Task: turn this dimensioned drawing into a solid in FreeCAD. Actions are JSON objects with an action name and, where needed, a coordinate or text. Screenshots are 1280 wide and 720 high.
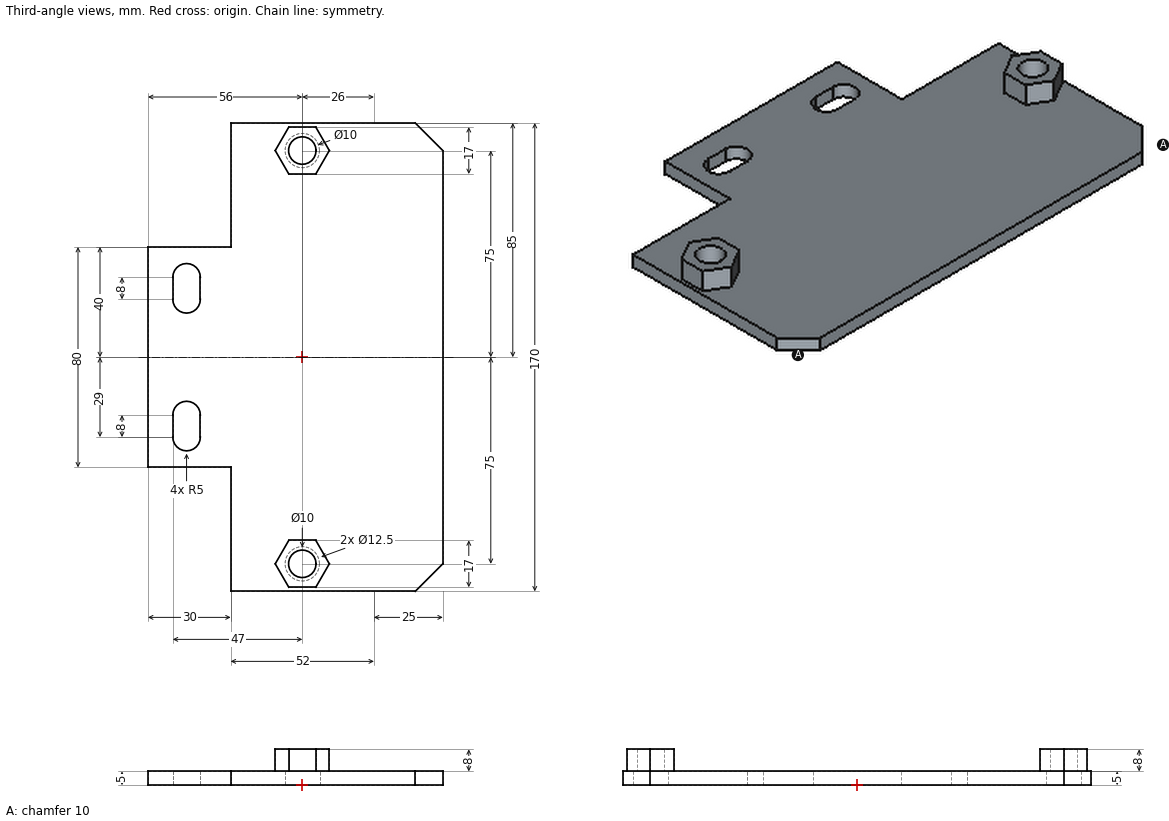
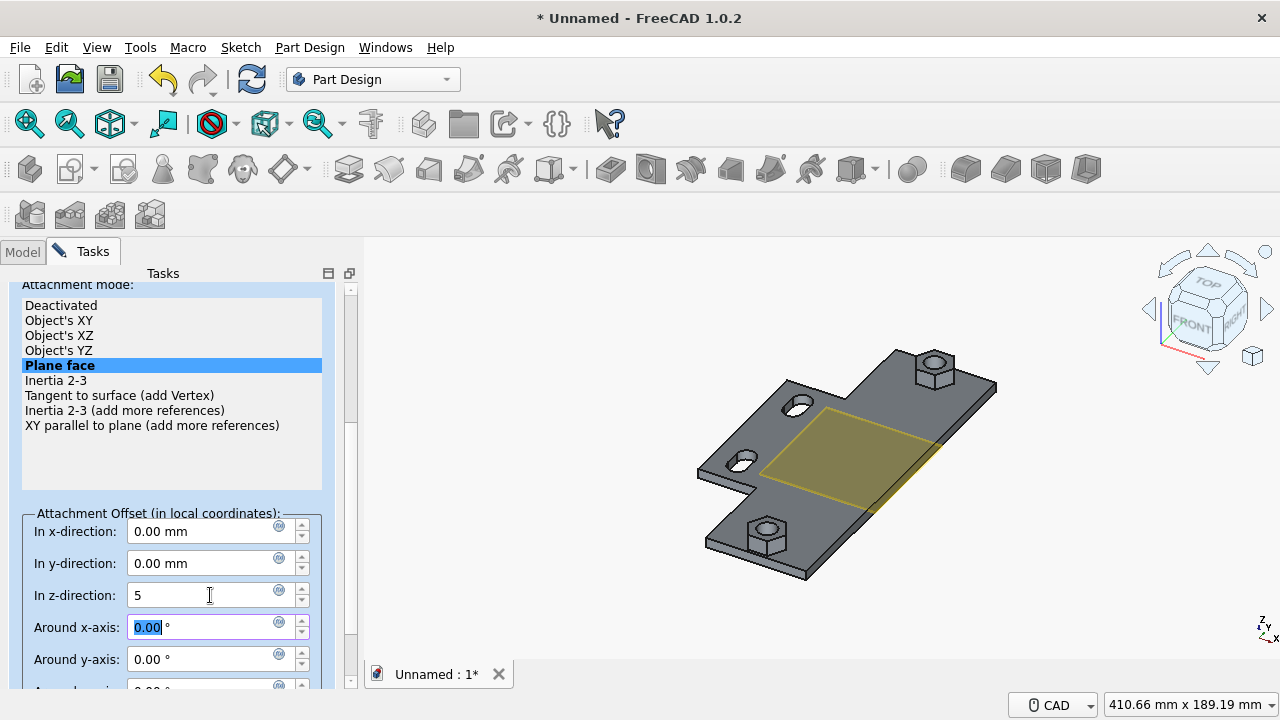
{"action": "scroll", "coordinate": [351, 486], "scroll_direction": "up", "scroll_amount": 5}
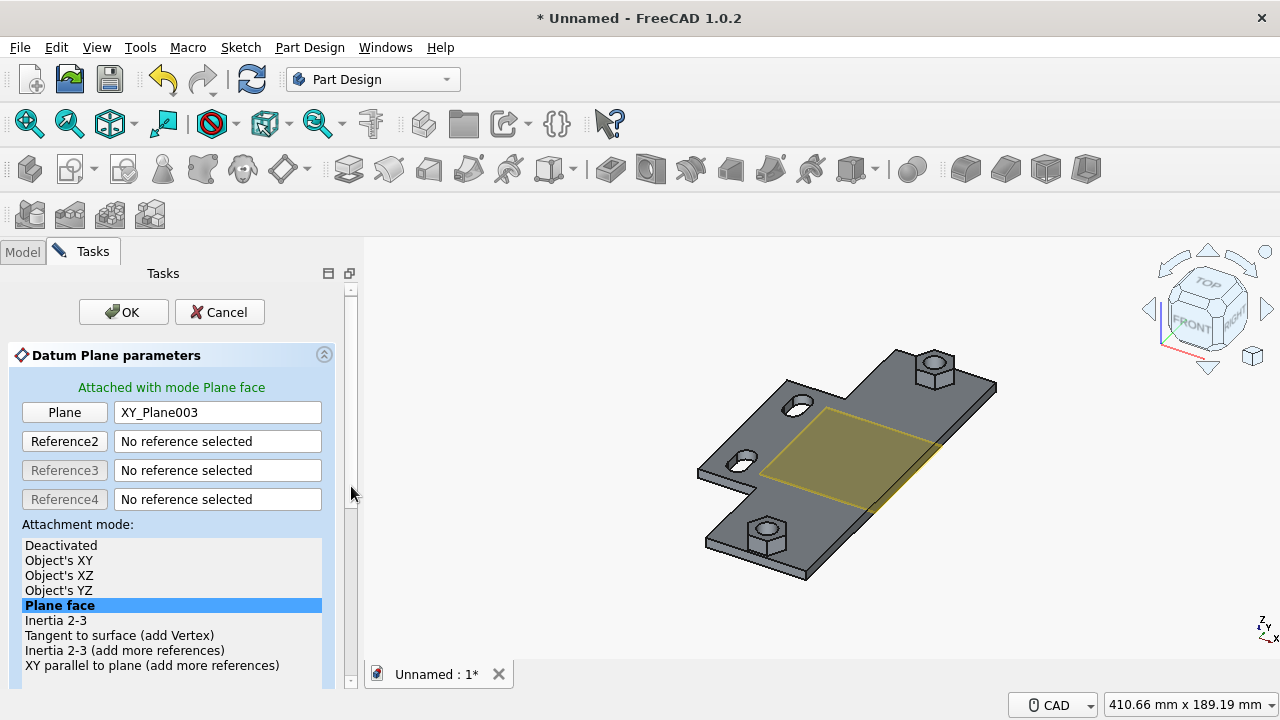
{"action": "left_click", "coordinate": [124, 312]}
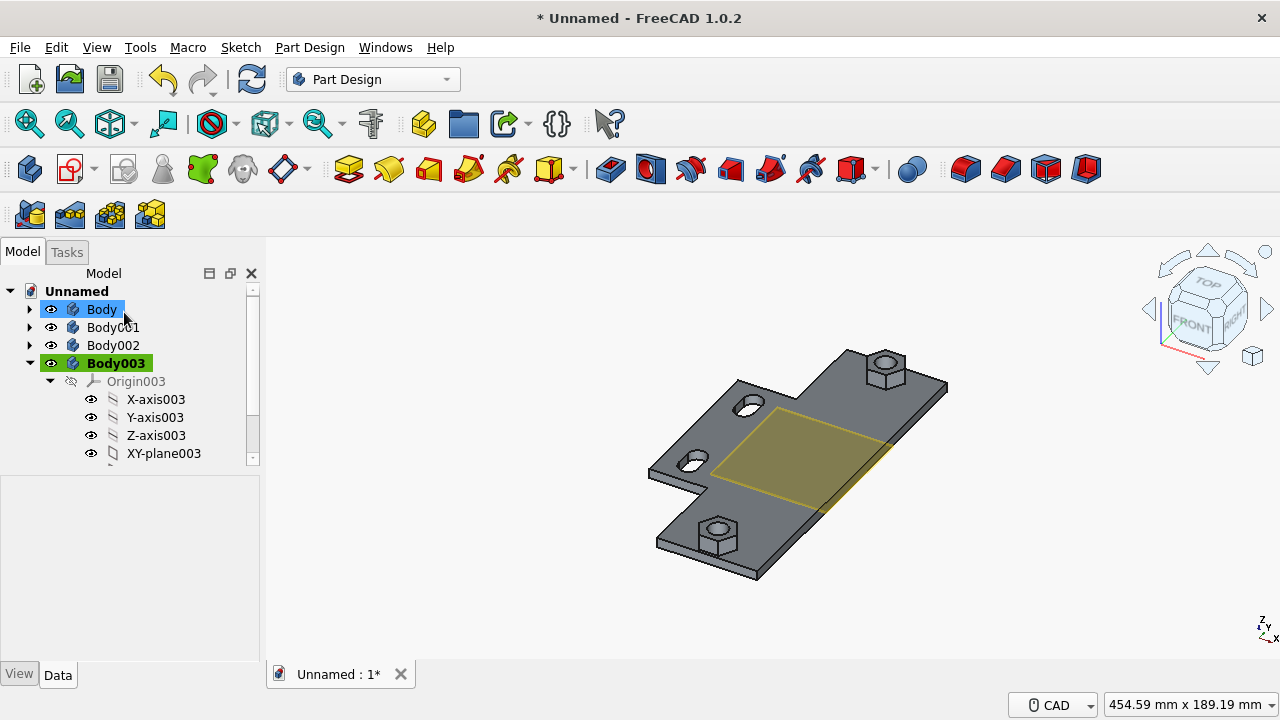
{"action": "scroll", "coordinate": [100, 377], "scroll_direction": "down", "scroll_amount": 3}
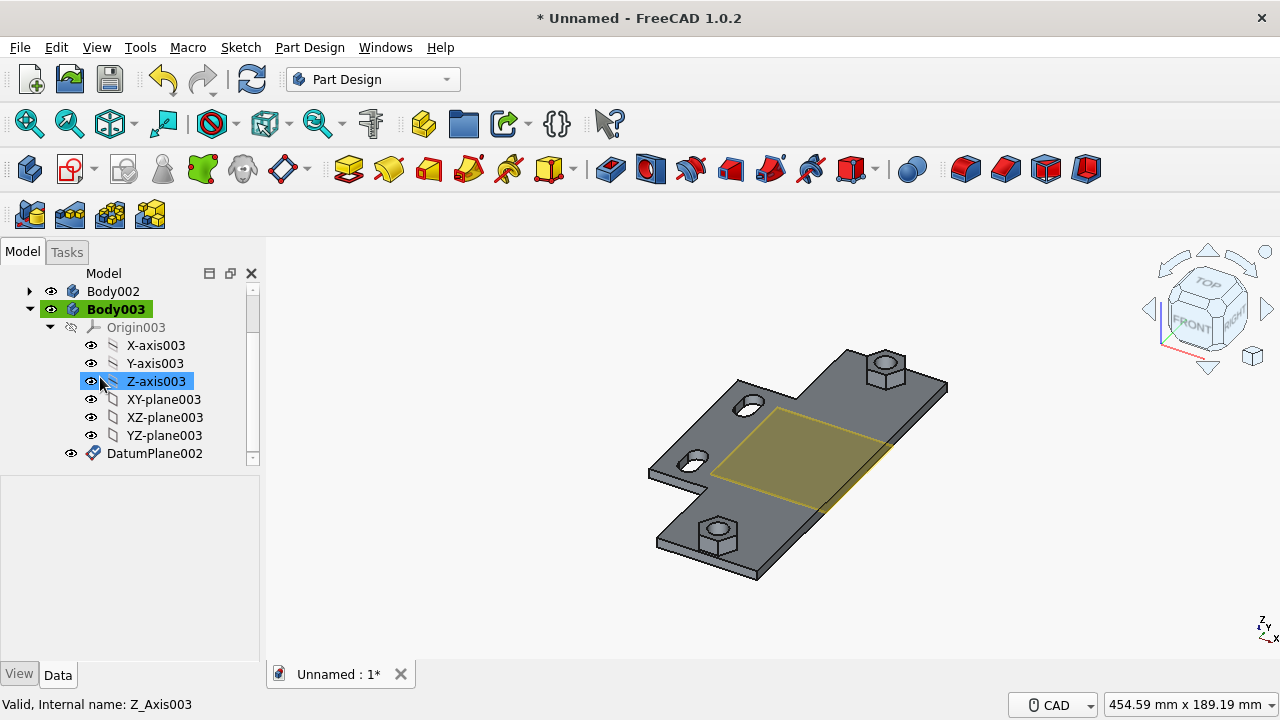
{"action": "left_click", "coordinate": [116, 453]}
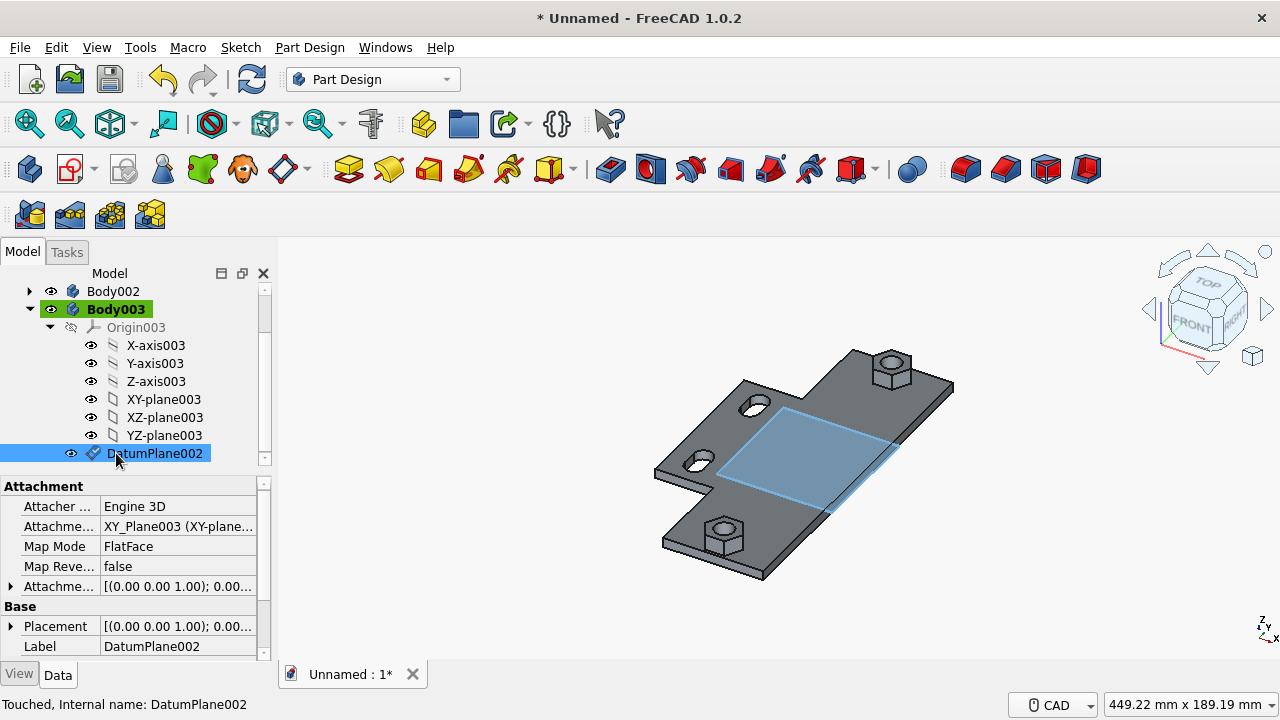
{"action": "left_click", "coordinate": [70, 170]}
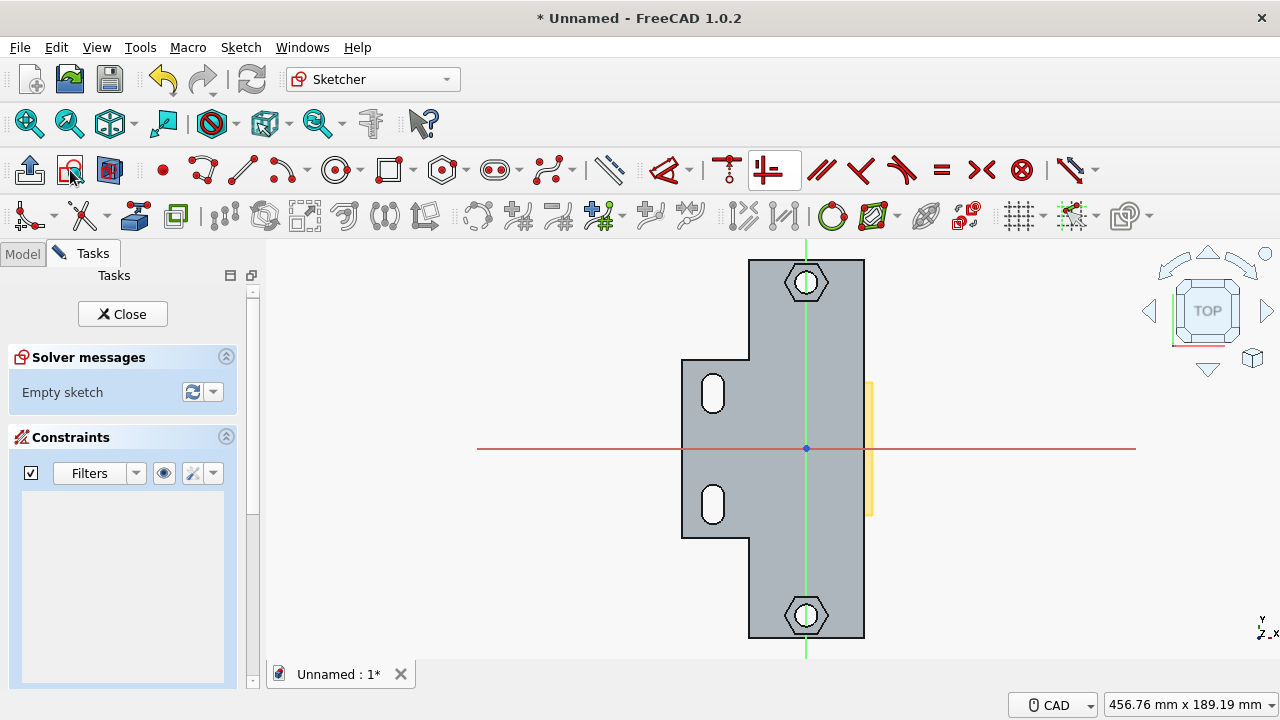
{"action": "scroll", "coordinate": [382, 449], "scroll_direction": "down", "scroll_amount": 2}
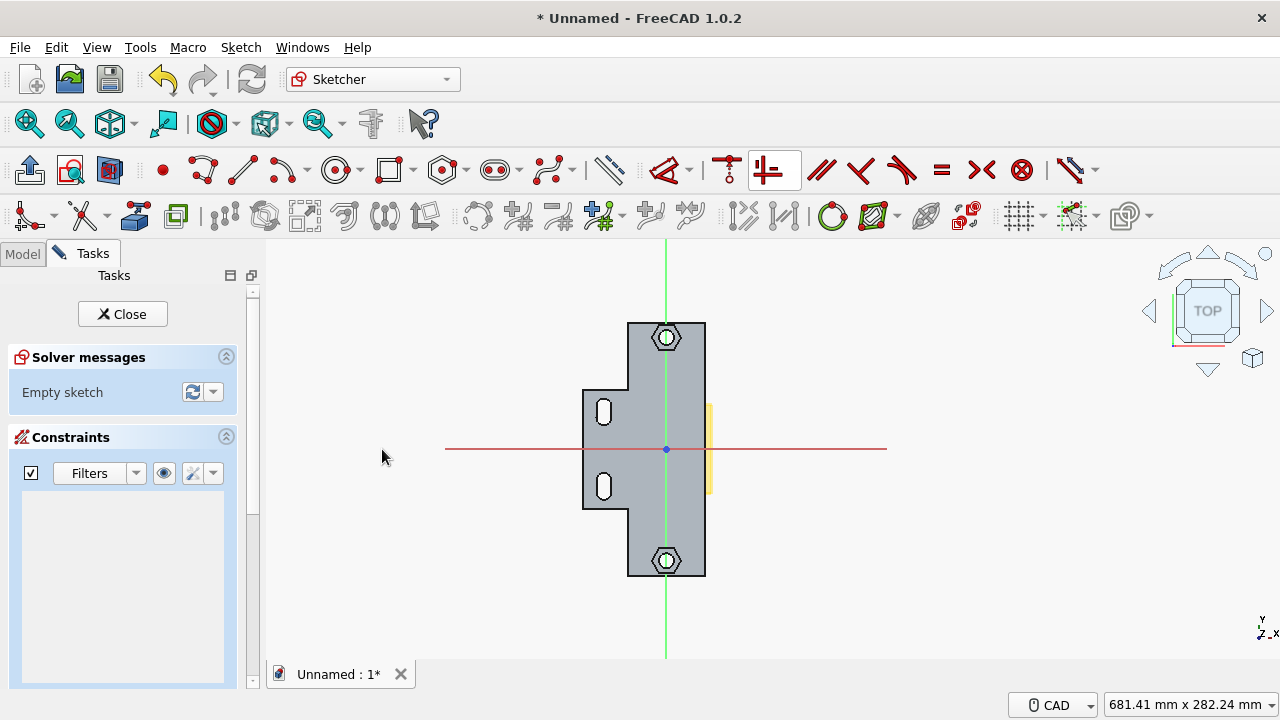
{"action": "left_click", "coordinate": [390, 170]}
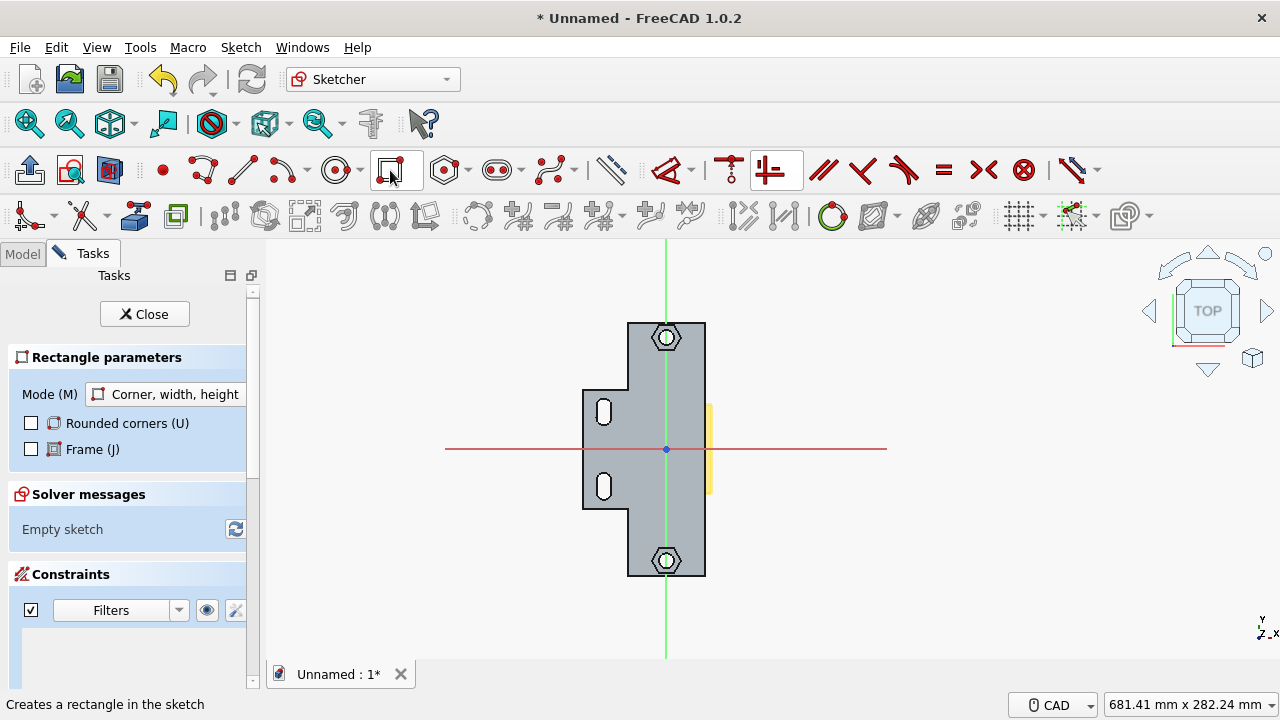
{"action": "left_click", "coordinate": [705, 323]}
{"action": "left_click", "coordinate": [742, 576]}
{"action": "key", "text": "Escape"}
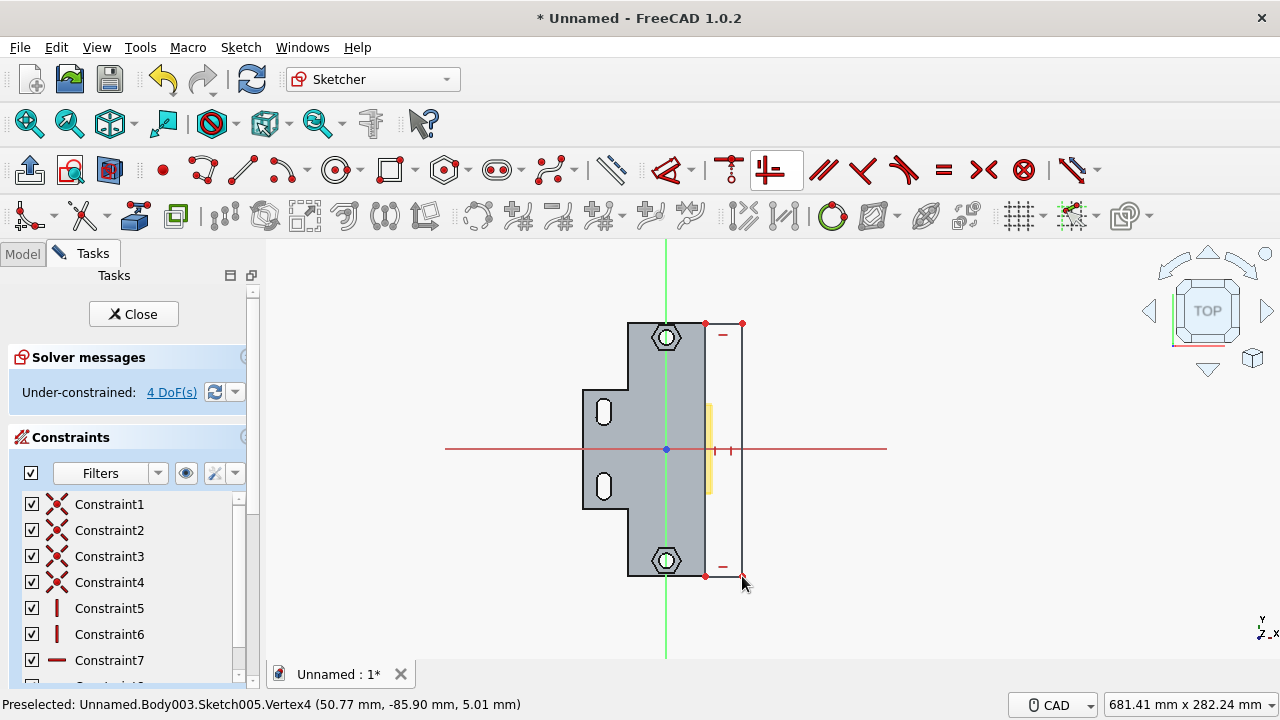
{"action": "left_click", "coordinate": [666, 170]}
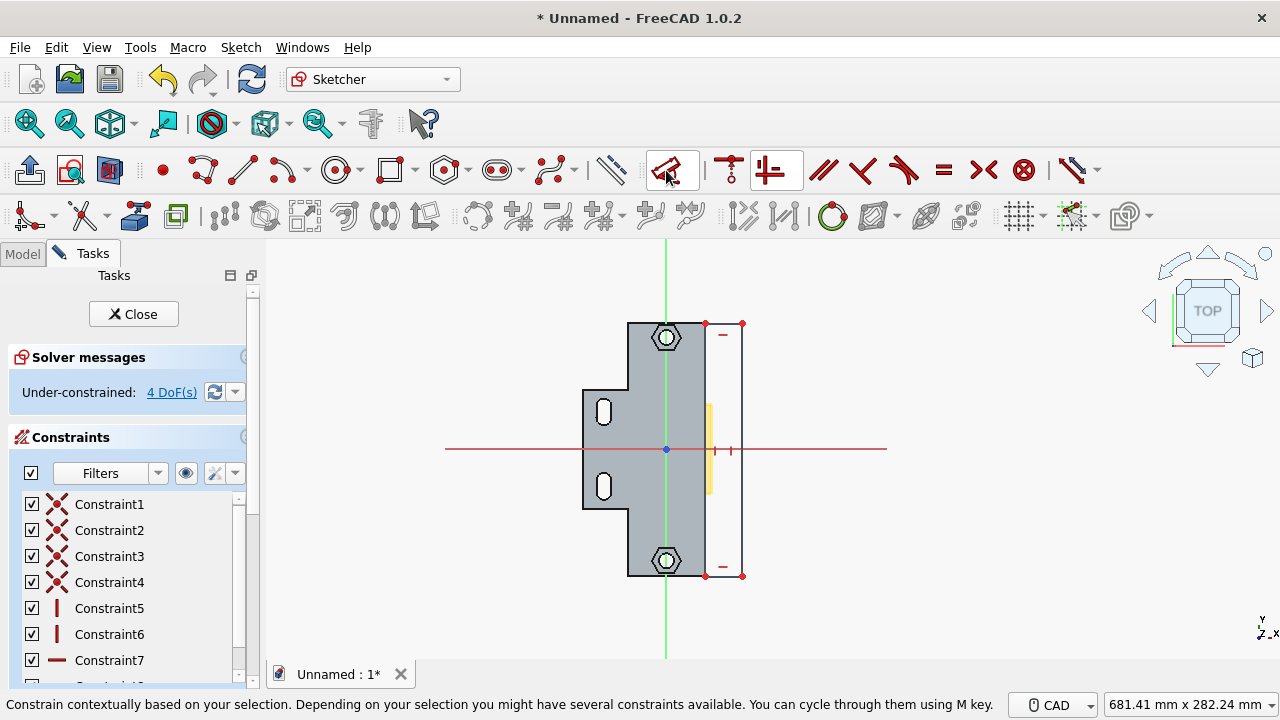
{"action": "scroll", "coordinate": [716, 577], "scroll_direction": "up", "scroll_amount": 2}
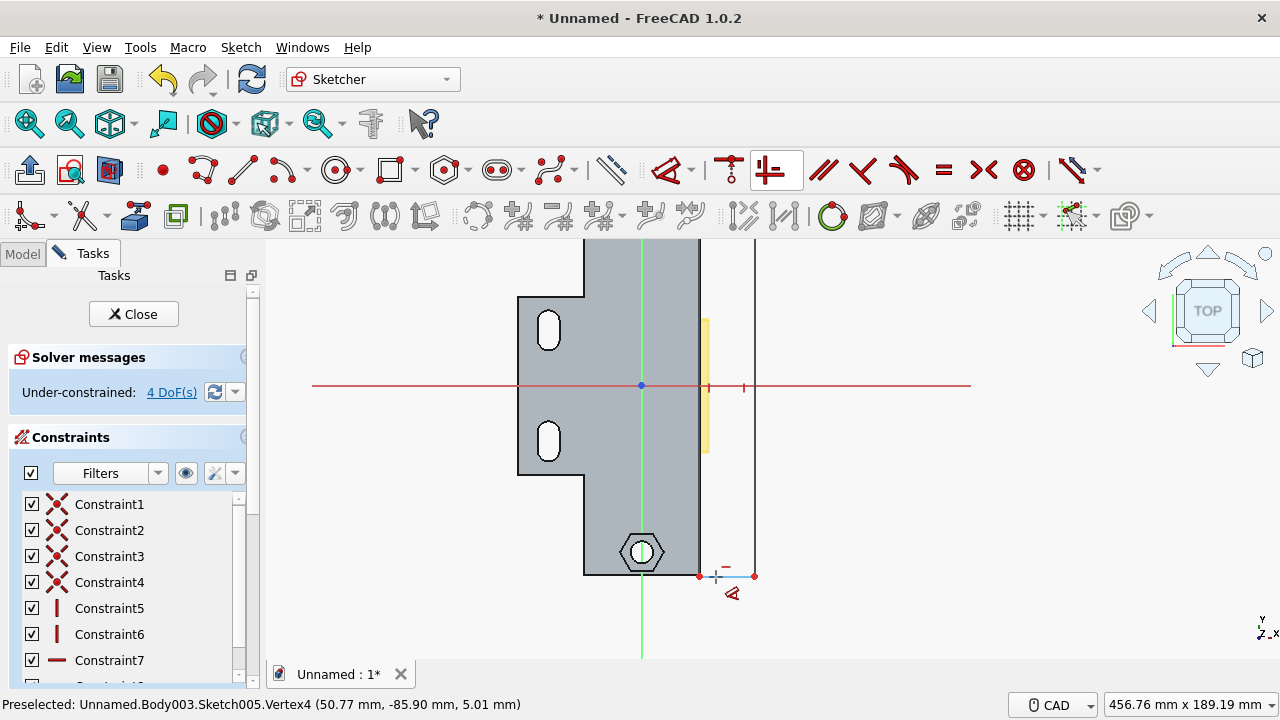
{"action": "left_click", "coordinate": [716, 577]}
{"action": "left_click", "coordinate": [727, 611]}